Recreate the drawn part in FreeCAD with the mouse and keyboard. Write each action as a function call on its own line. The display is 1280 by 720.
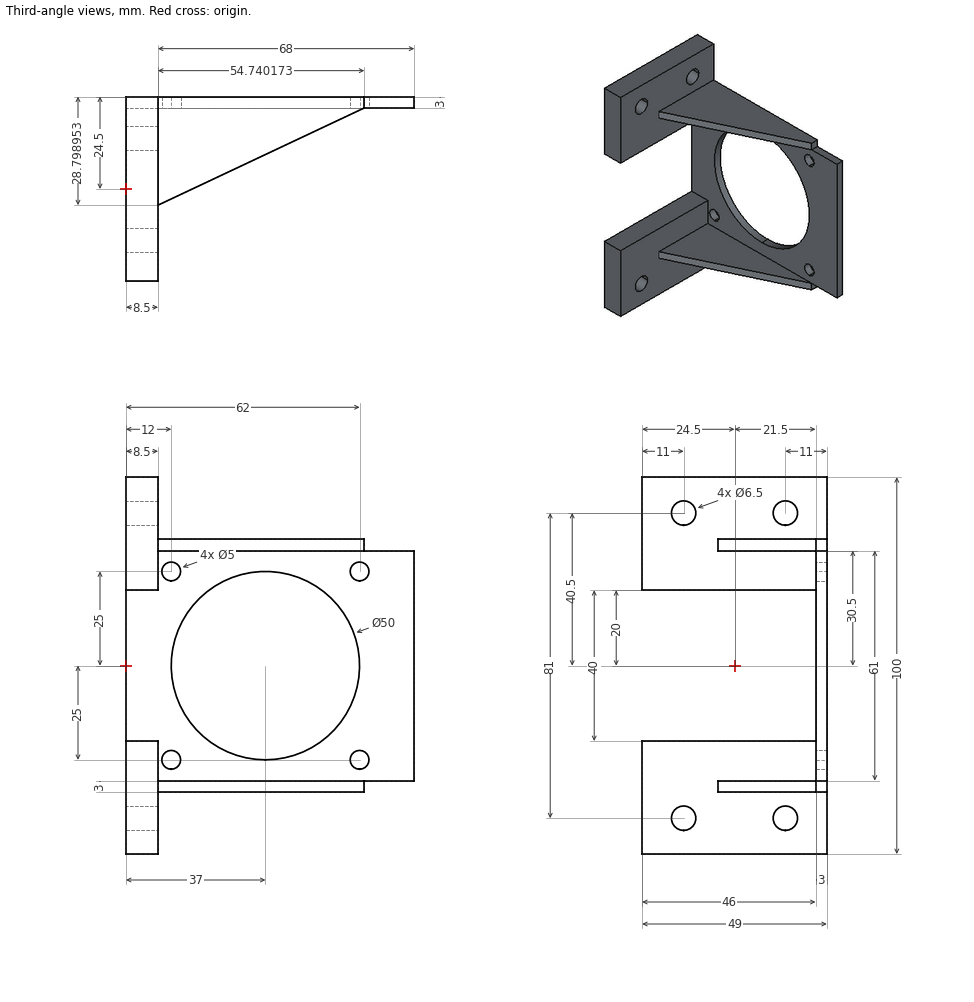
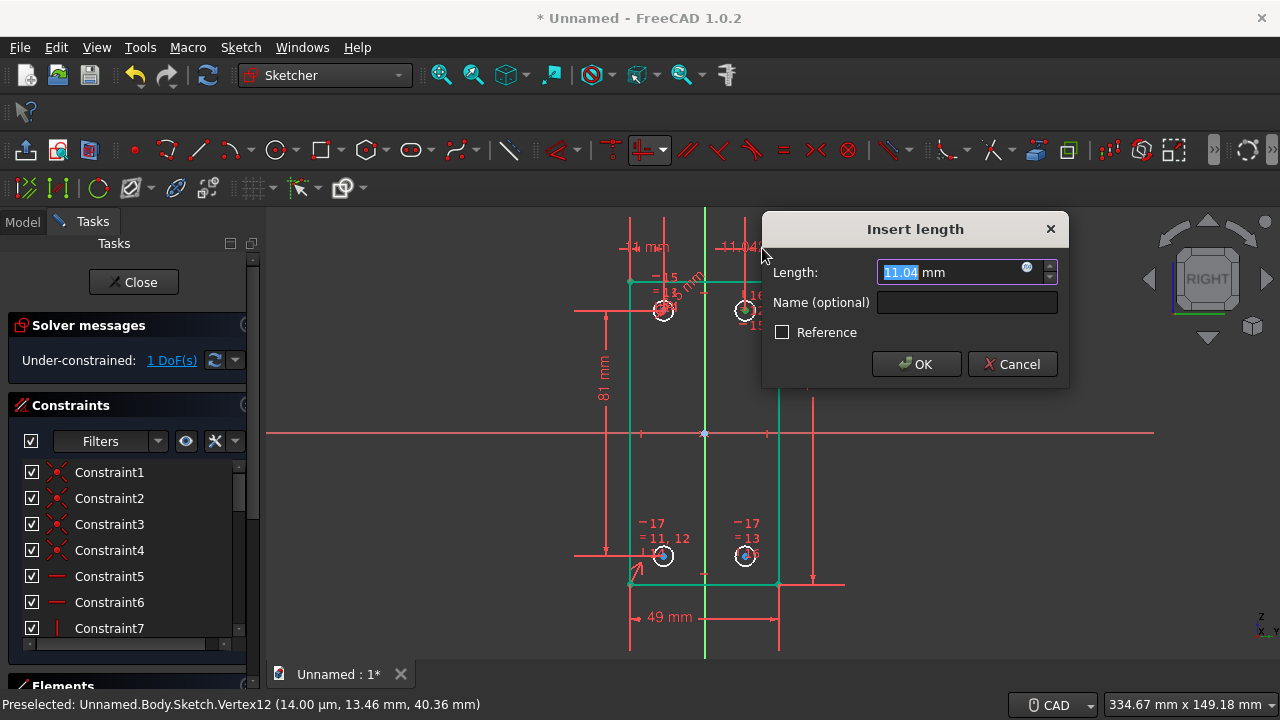
text(11)
key(Return)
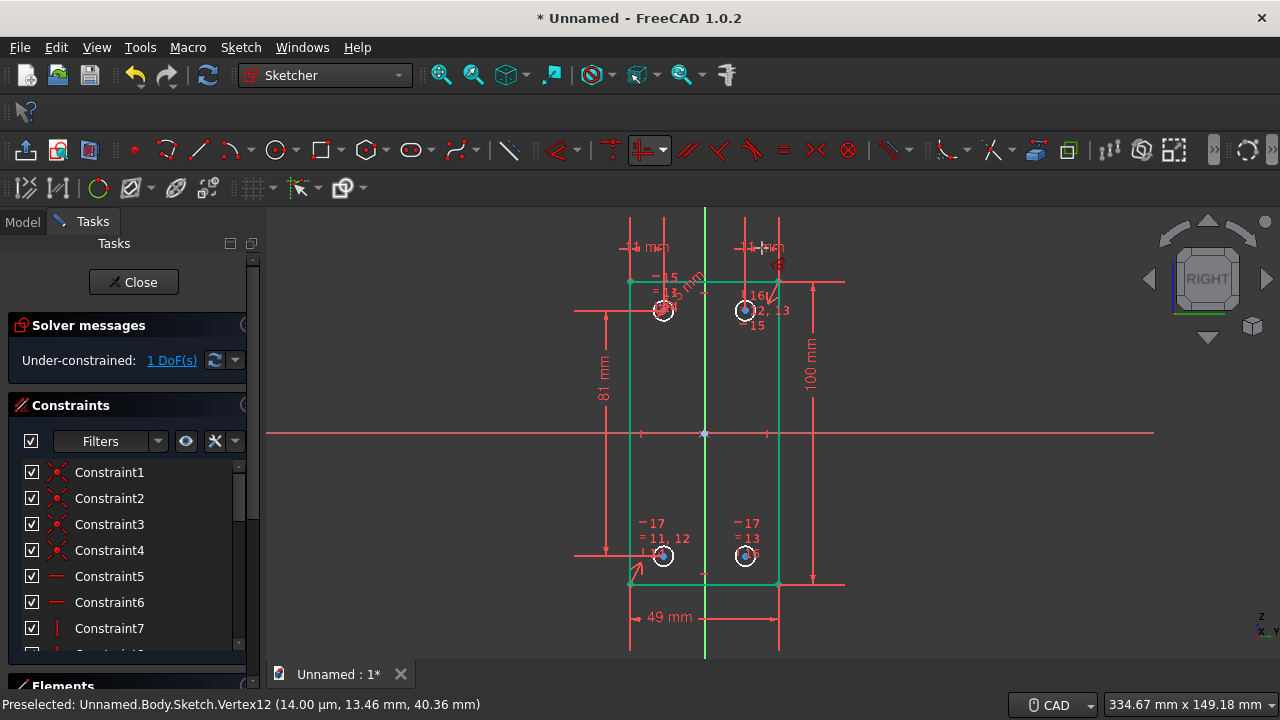
click(664, 311)
click(739, 372)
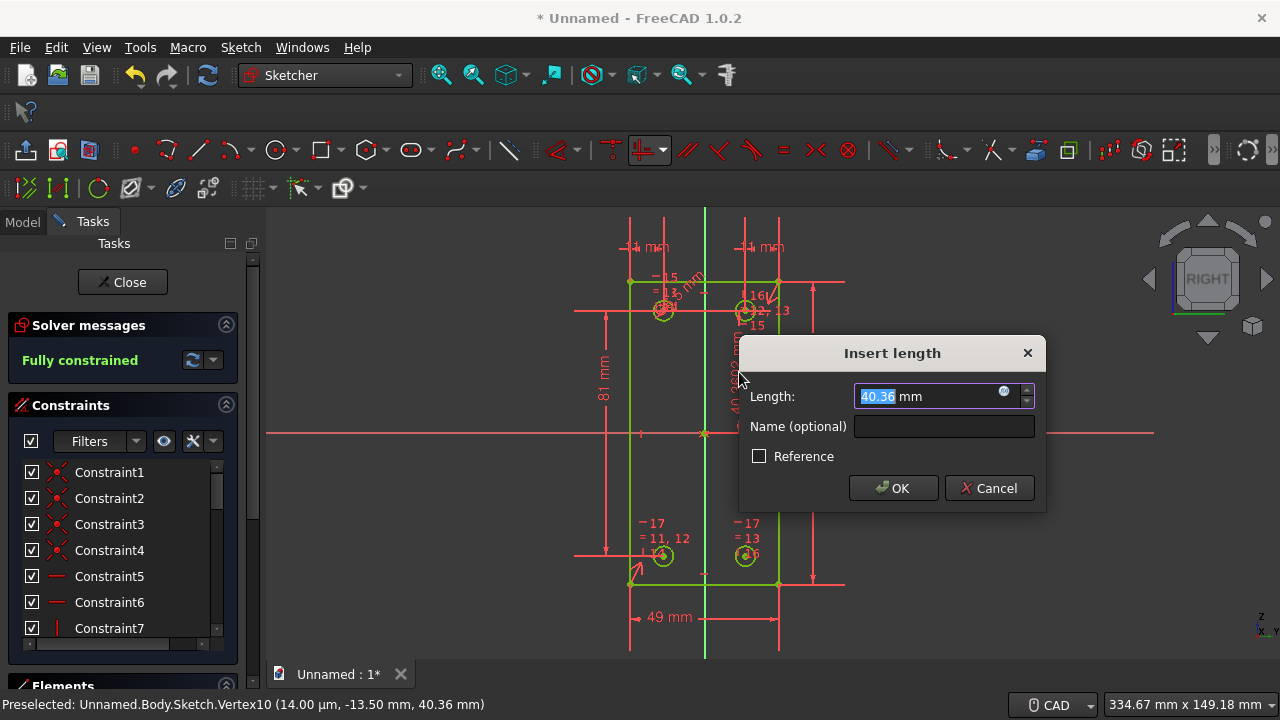
text(40.5)
key(Return)
key(Escape)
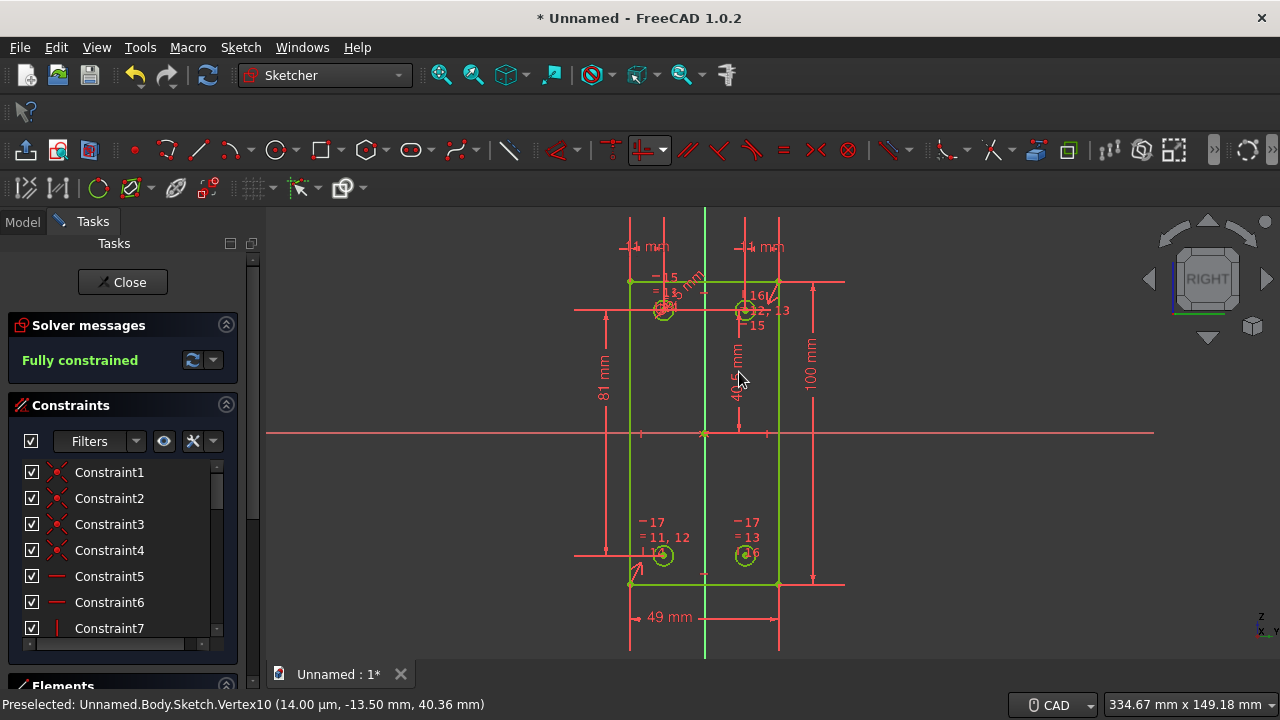
click(123, 282)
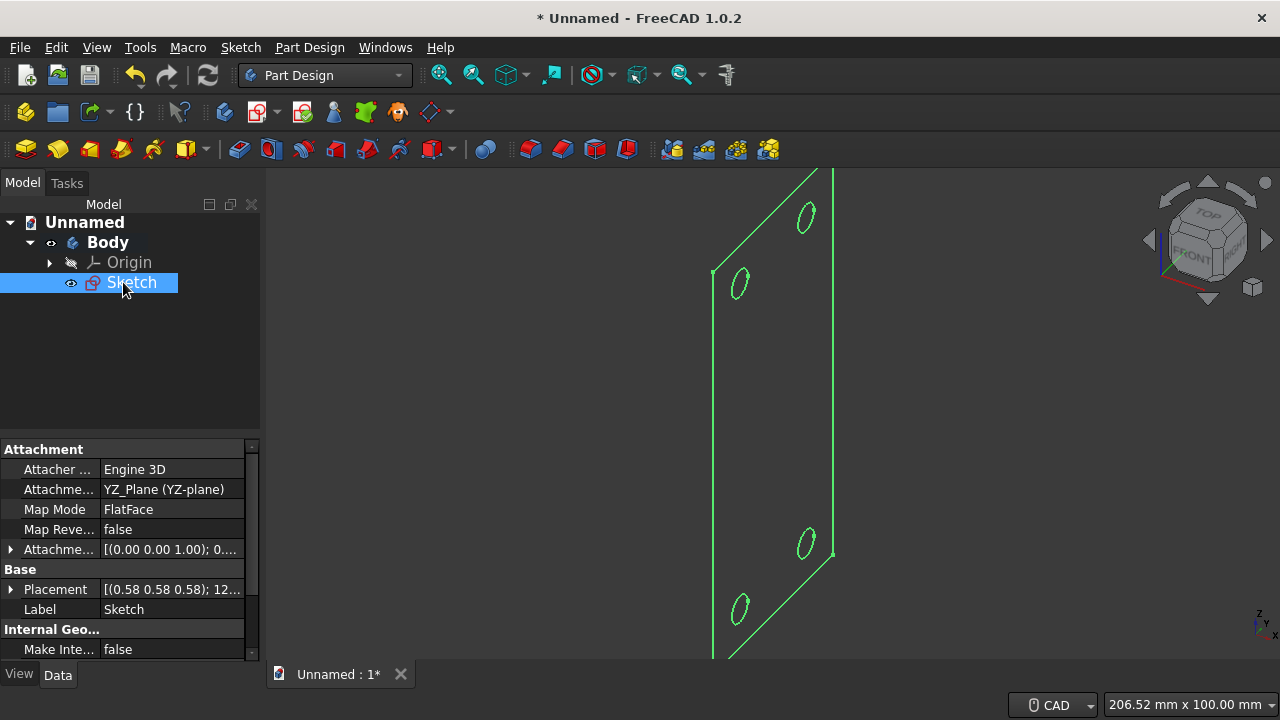
click(26, 150)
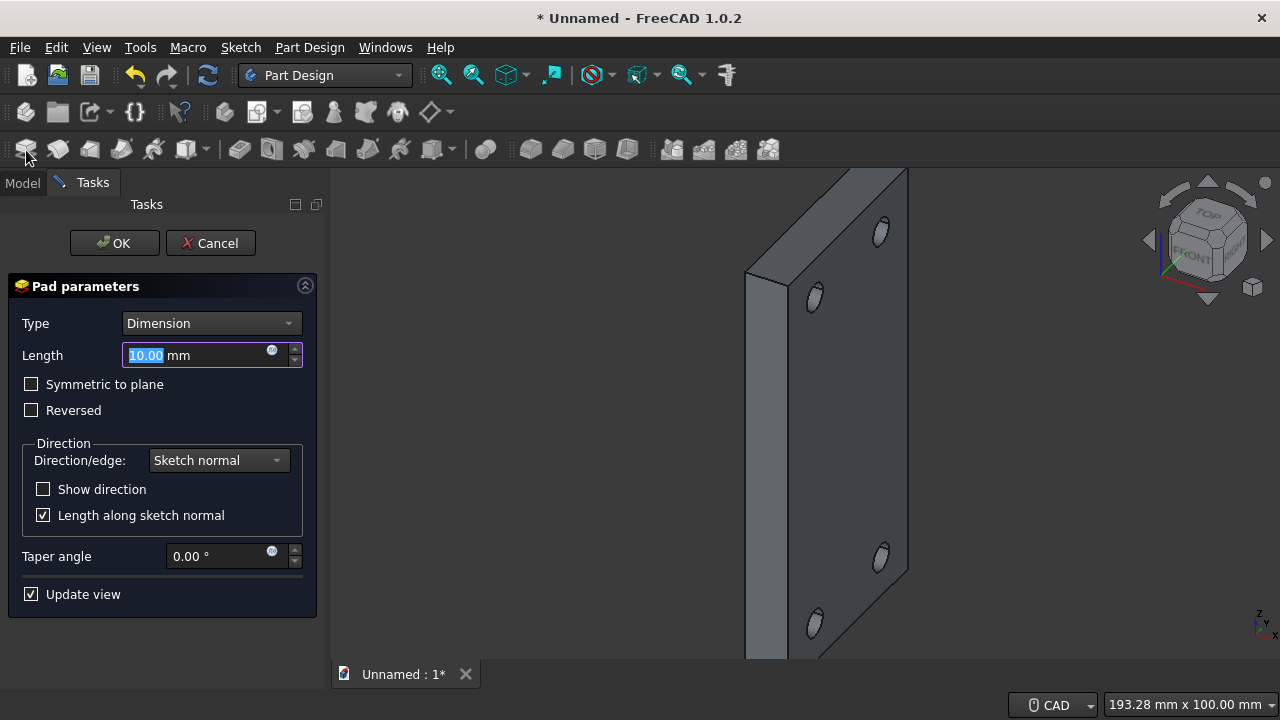
text(8.5)
key(Tab)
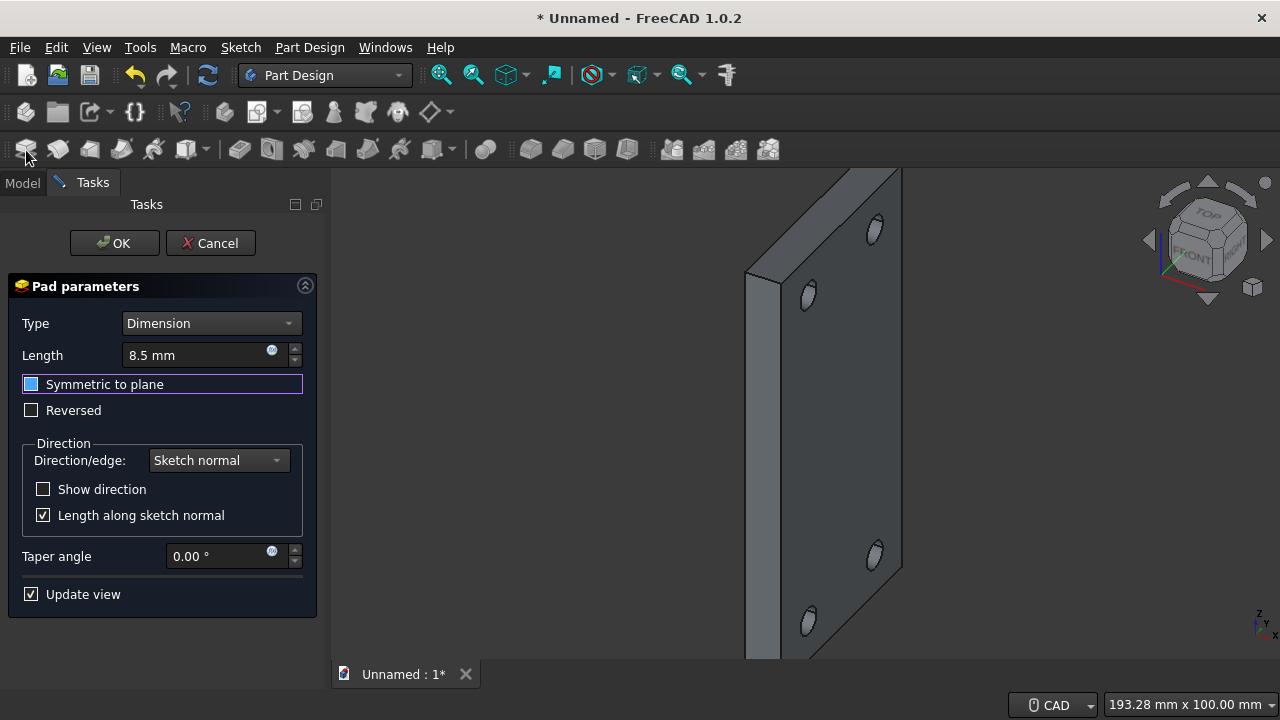
click(115, 243)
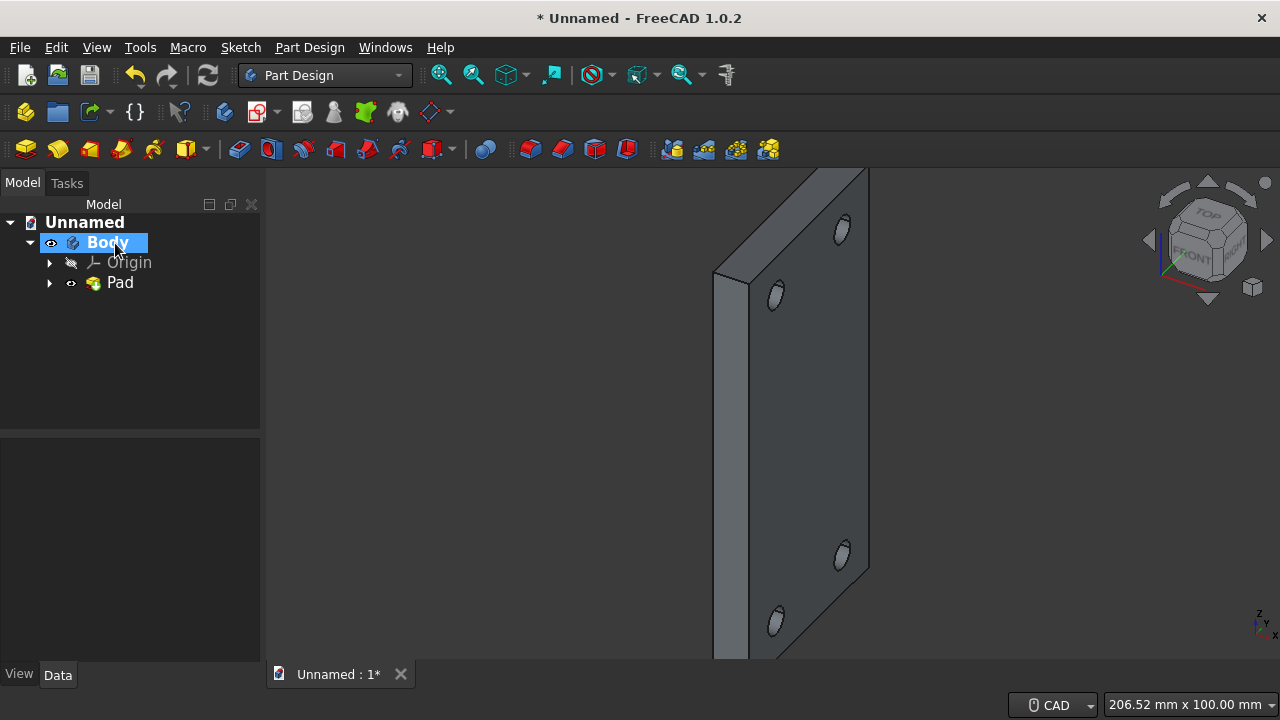
key(v)
key(f)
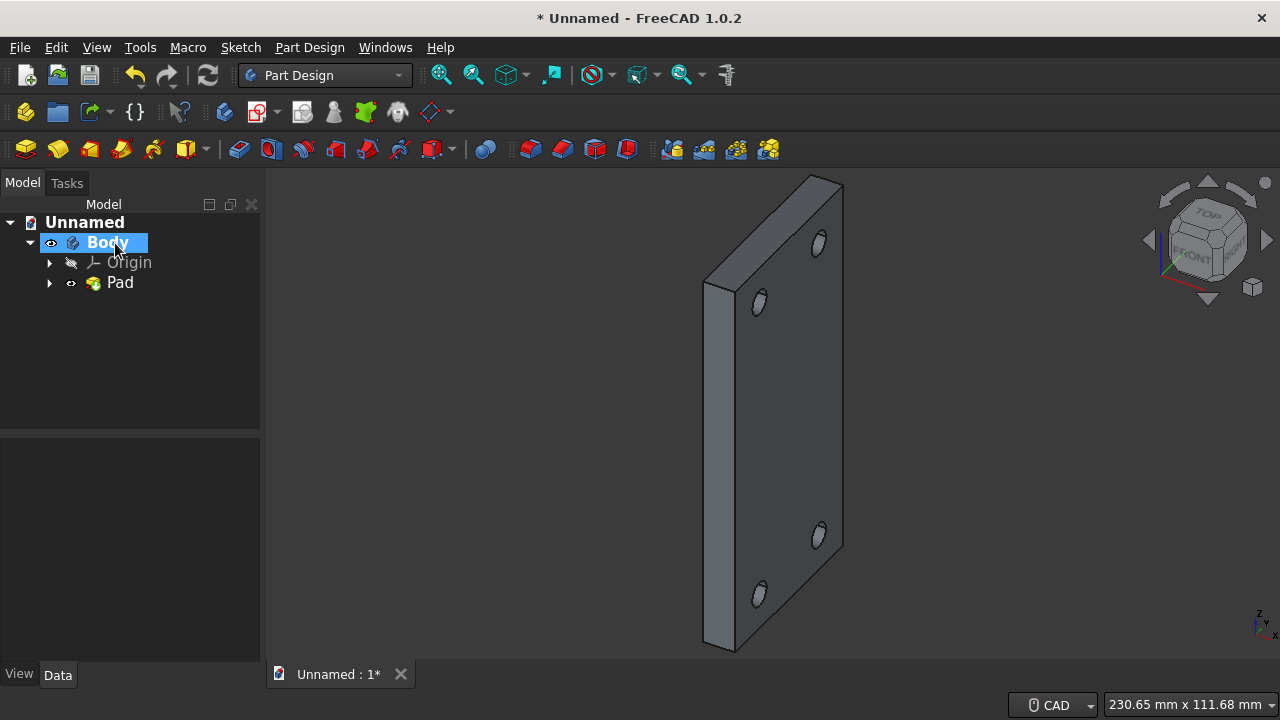
click(789, 418)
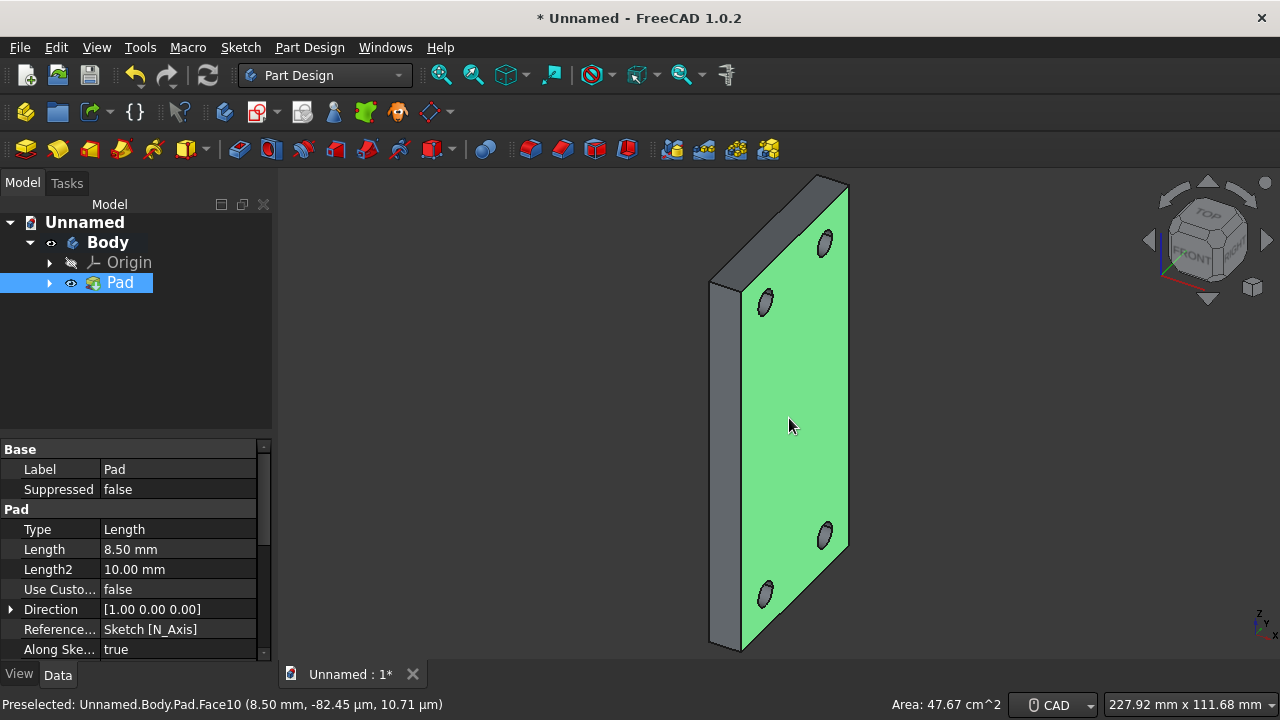
click(258, 112)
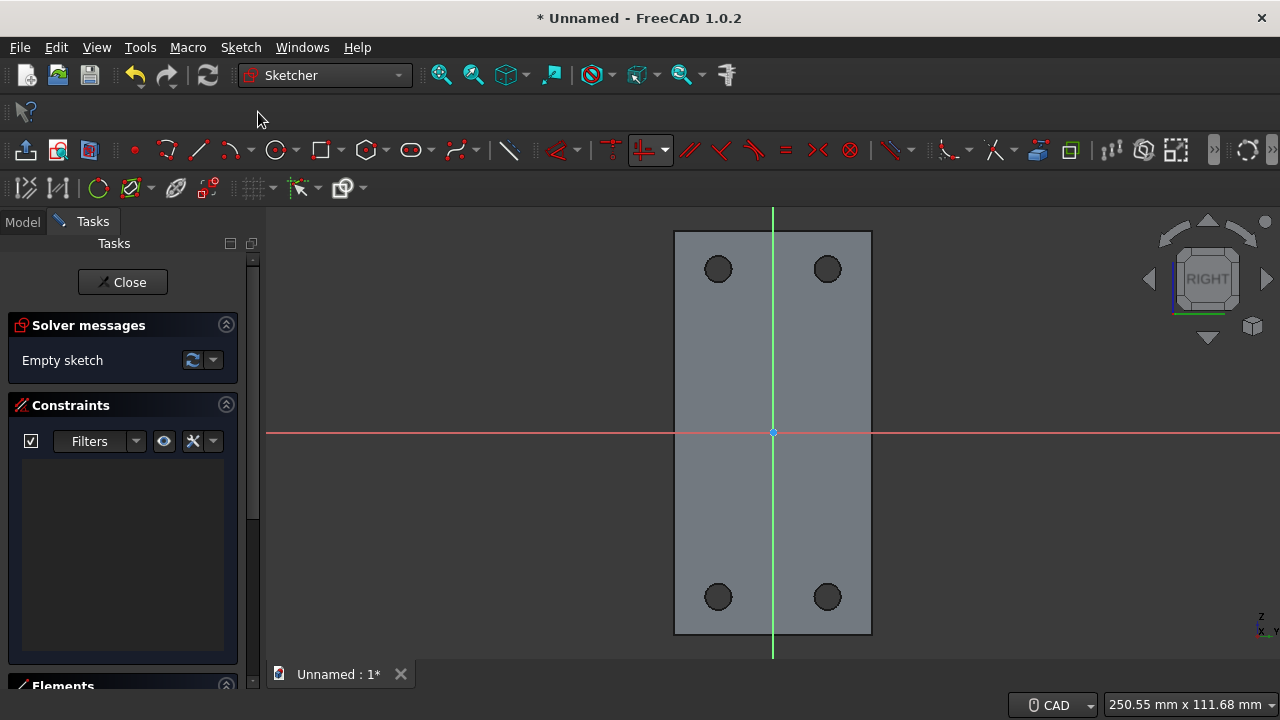
click(322, 150)